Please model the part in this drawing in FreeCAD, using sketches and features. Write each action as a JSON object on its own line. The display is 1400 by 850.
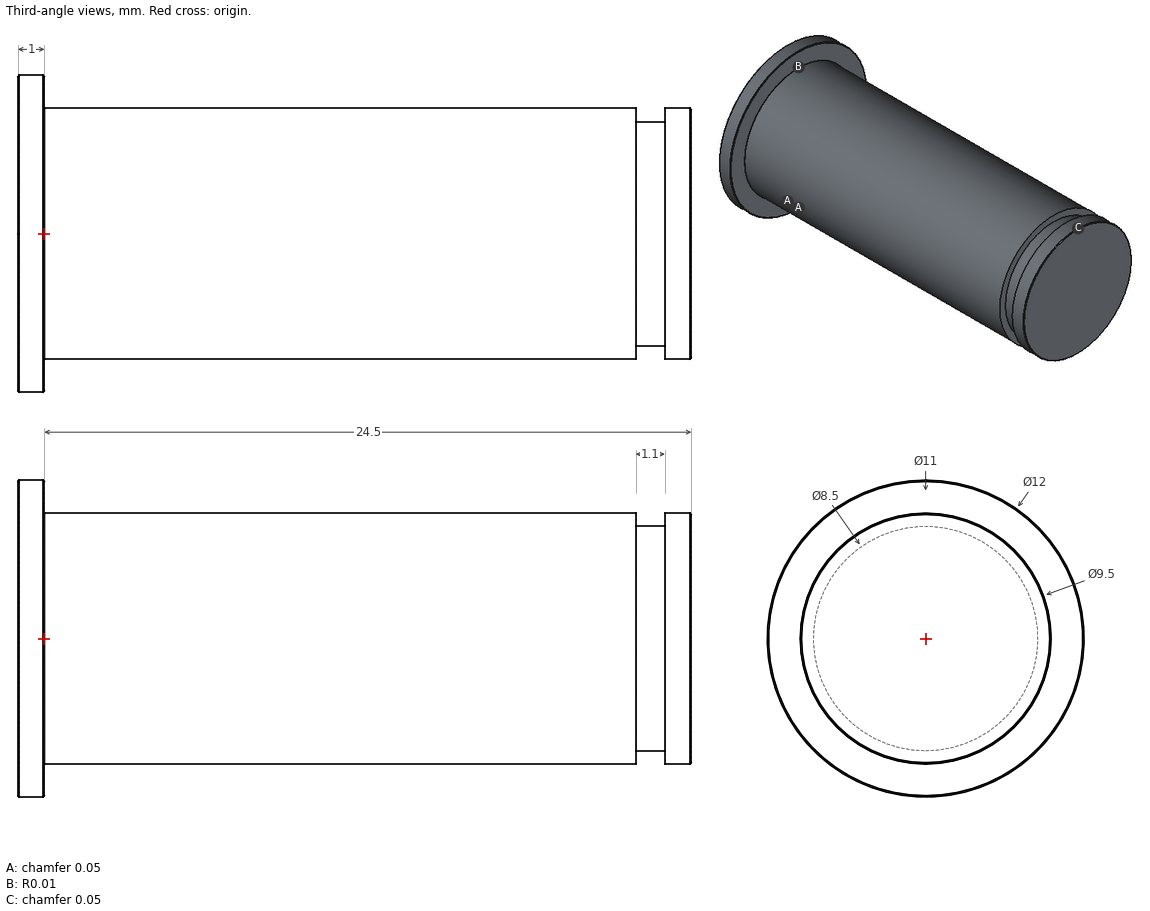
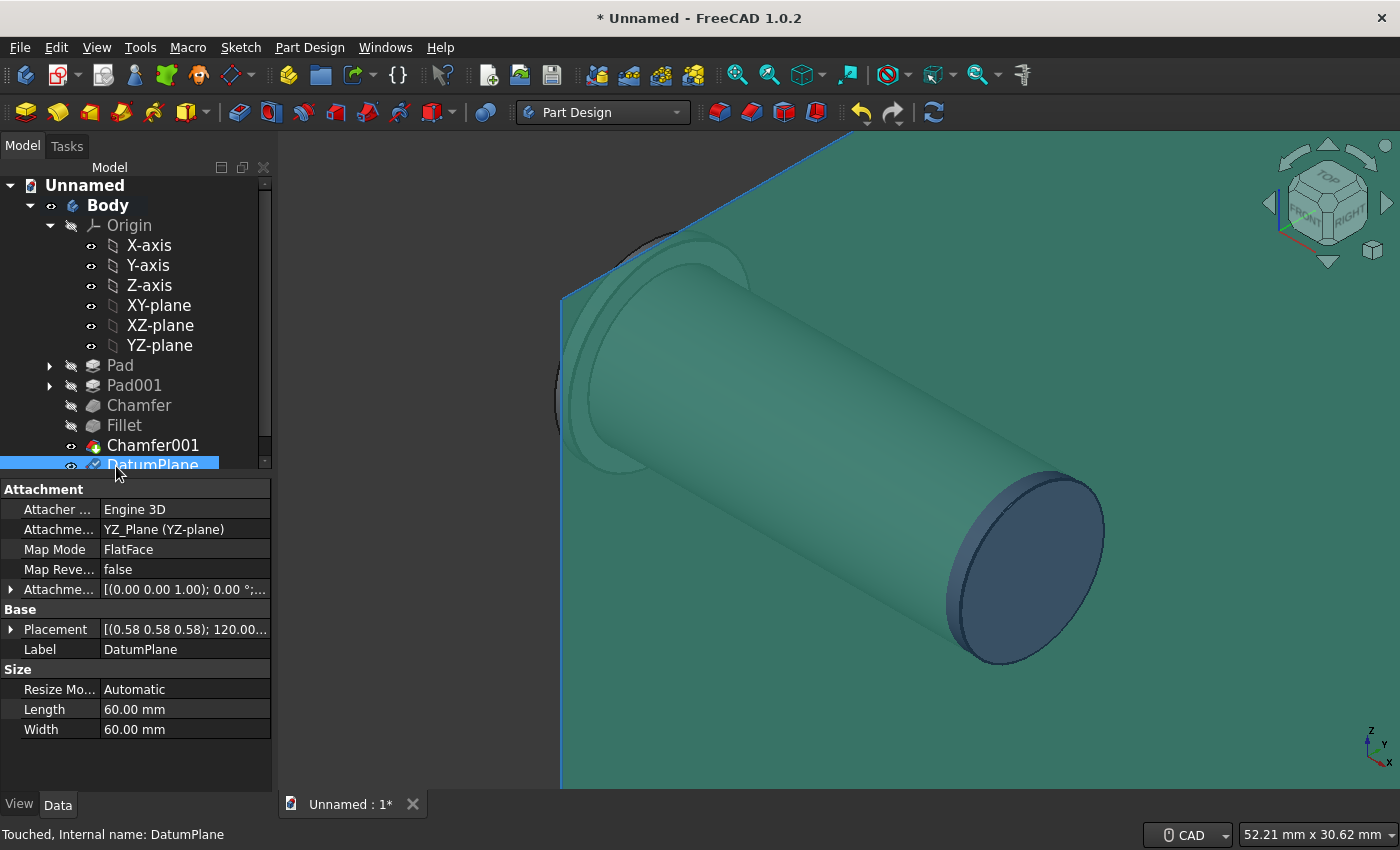
{"action": "left_click", "coordinate": [58, 76]}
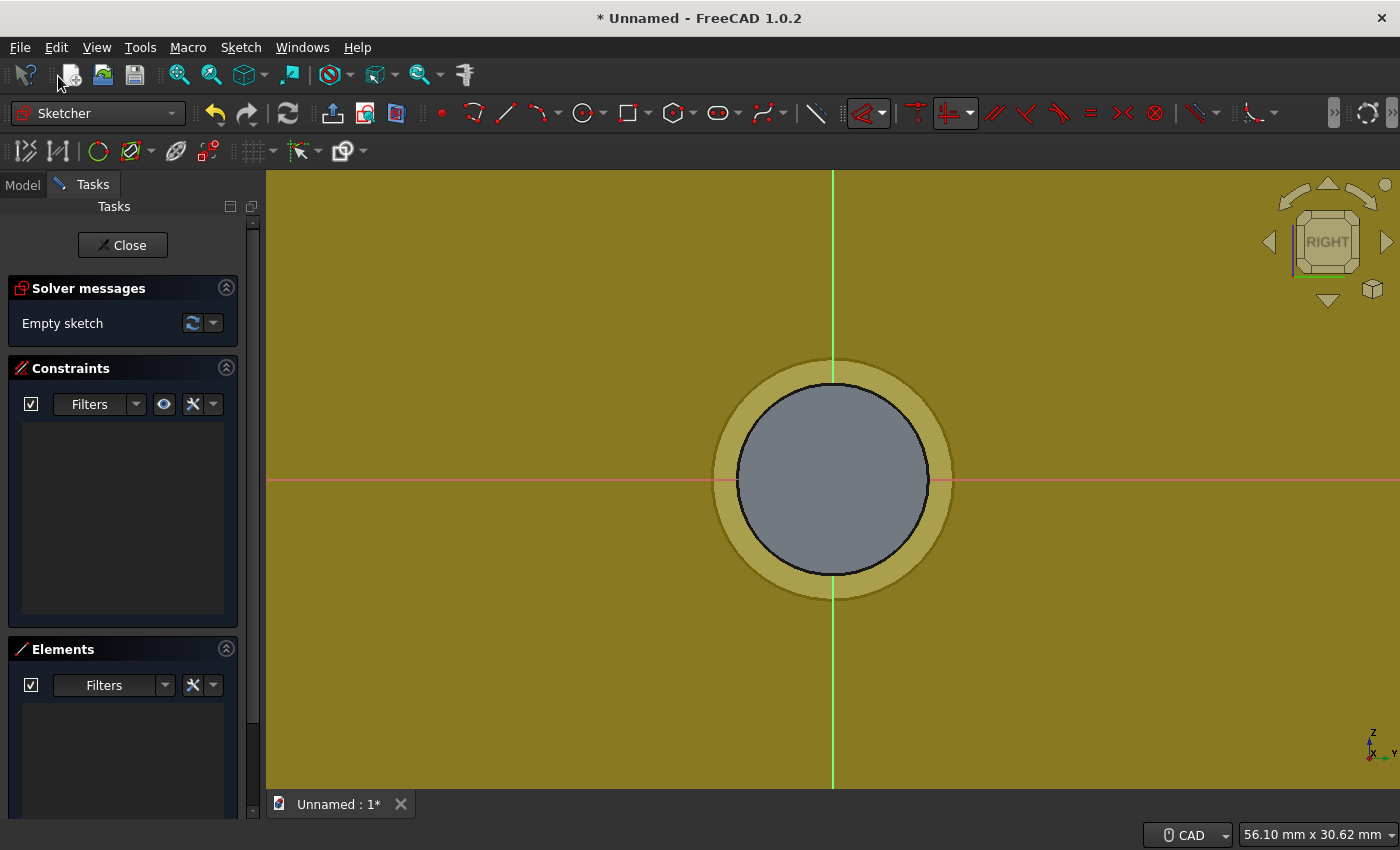
{"action": "left_click", "coordinate": [398, 114]}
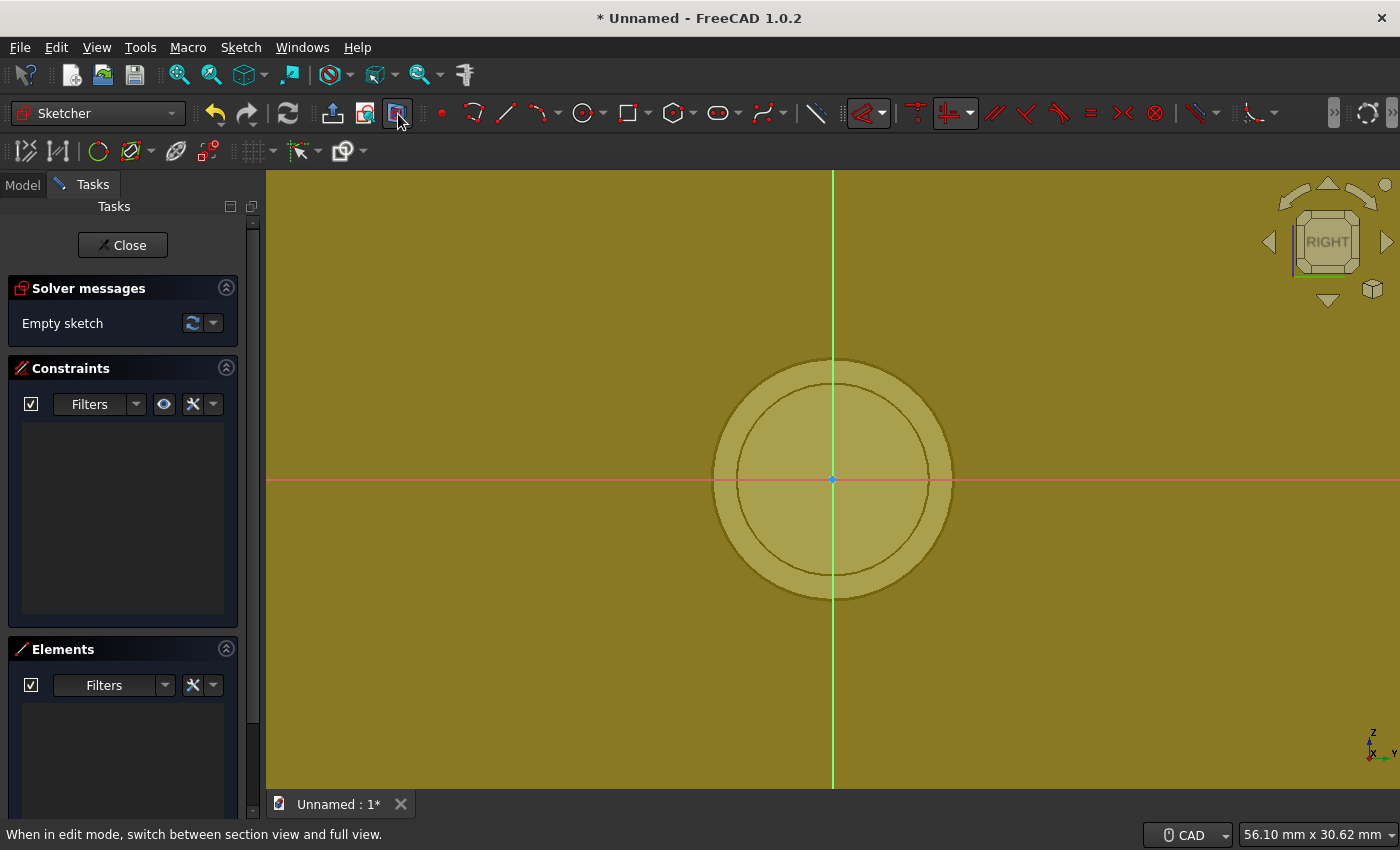
{"action": "scroll", "coordinate": [916, 480], "scroll_direction": "up", "scroll_amount": 3}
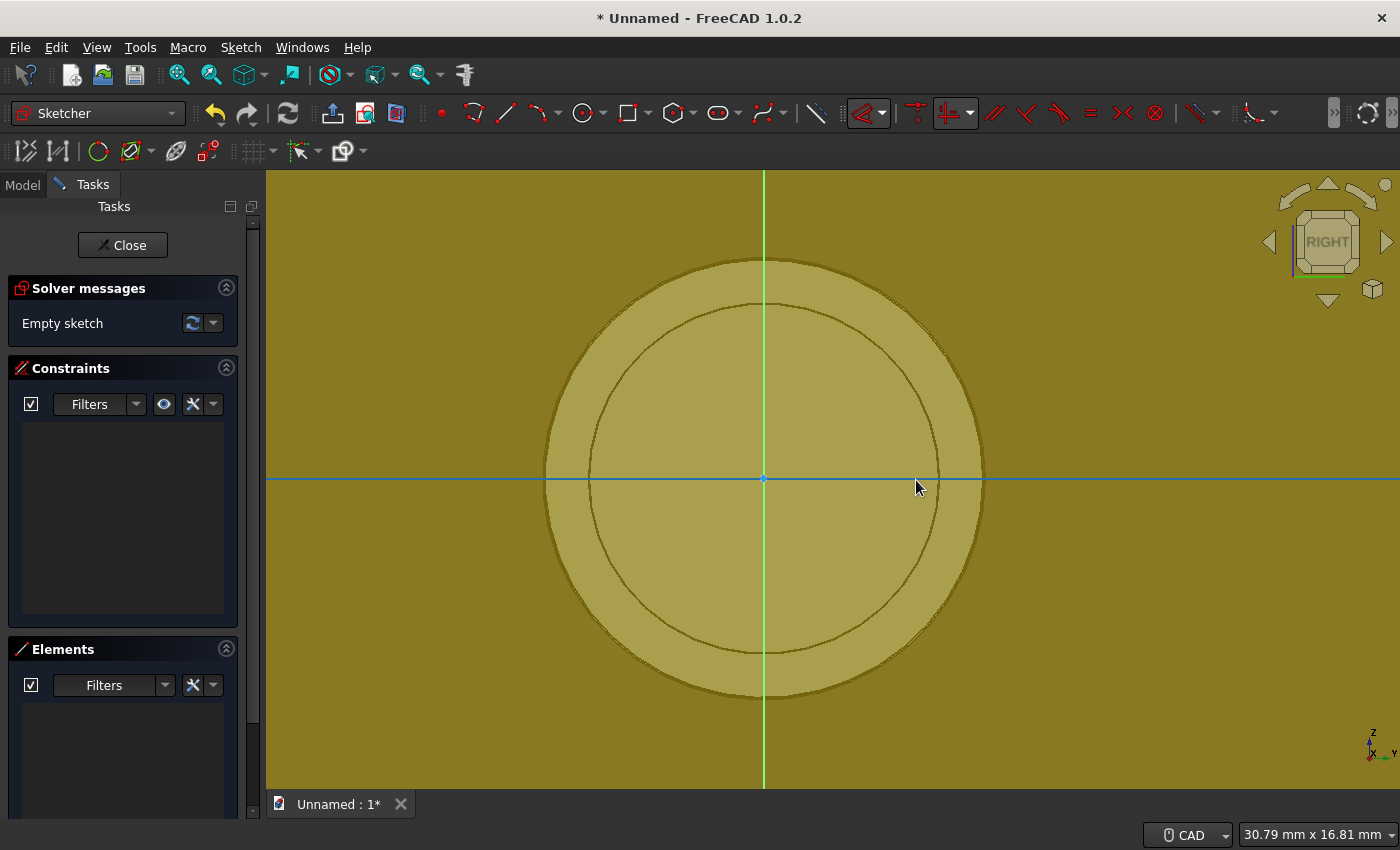
{"action": "left_click", "coordinate": [584, 114]}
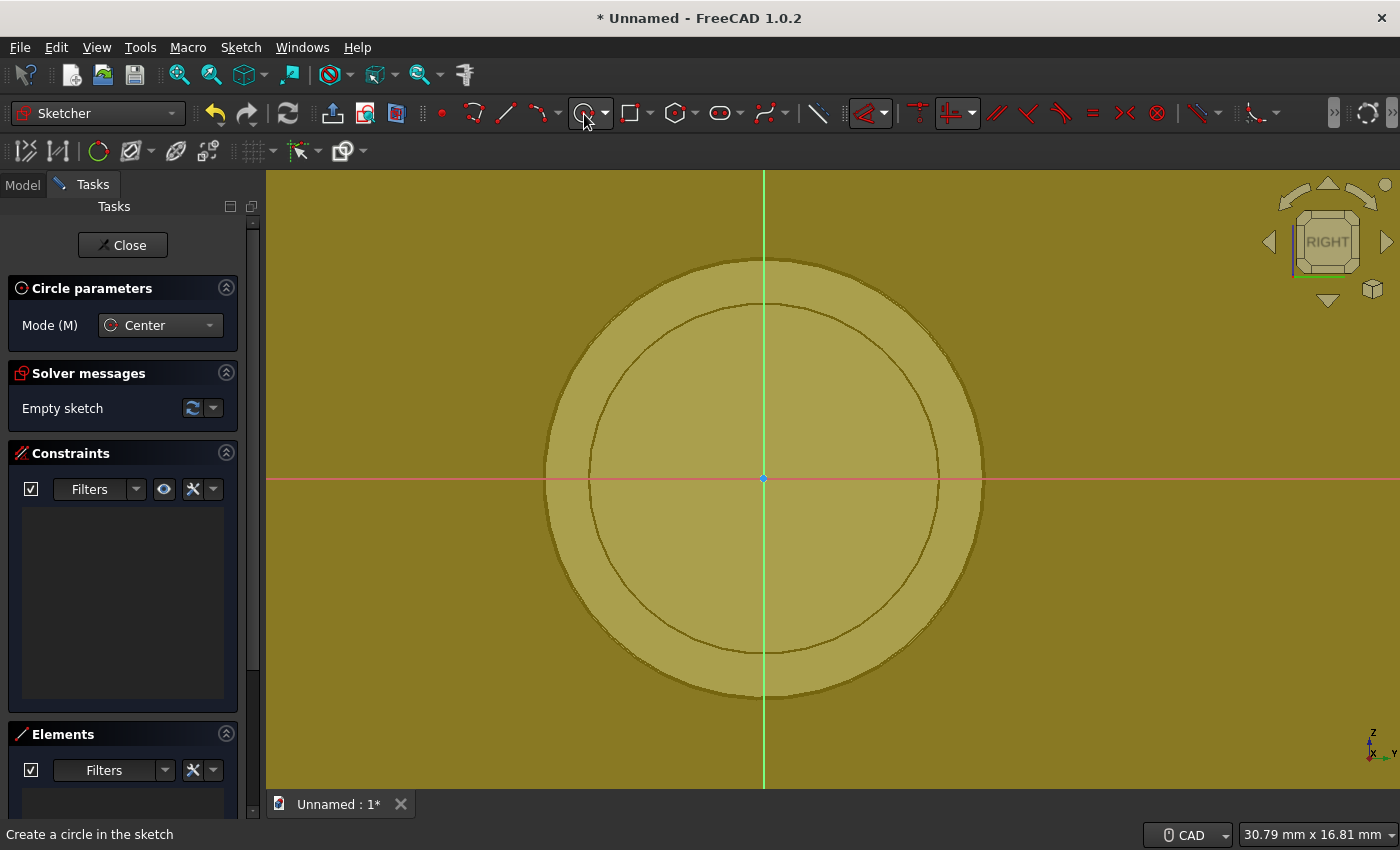
{"action": "left_click", "coordinate": [764, 479]}
{"action": "left_click", "coordinate": [907, 335]}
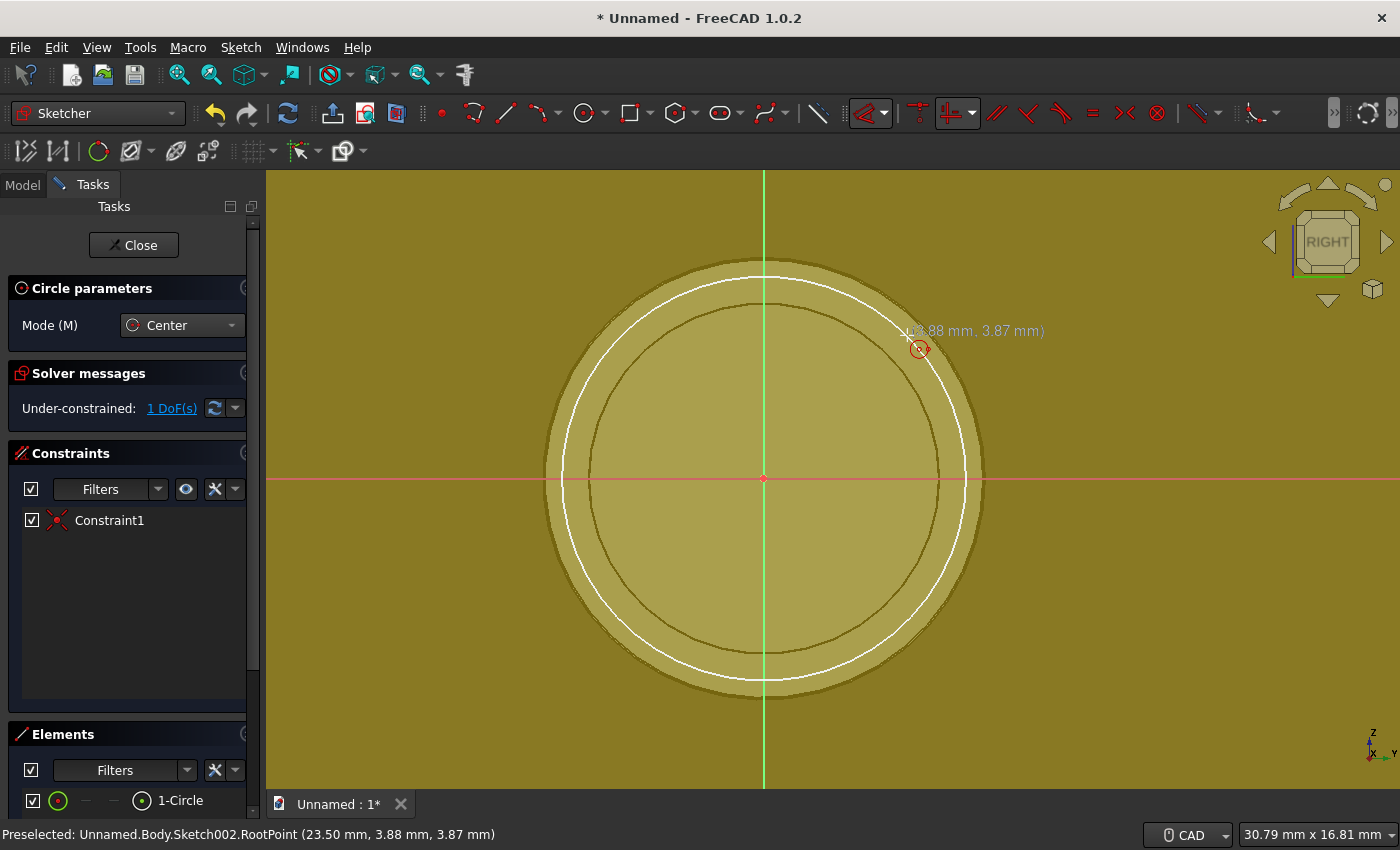
{"action": "left_click", "coordinate": [764, 479]}
{"action": "left_click", "coordinate": [875, 368]}
{"action": "key", "text": "Escape"}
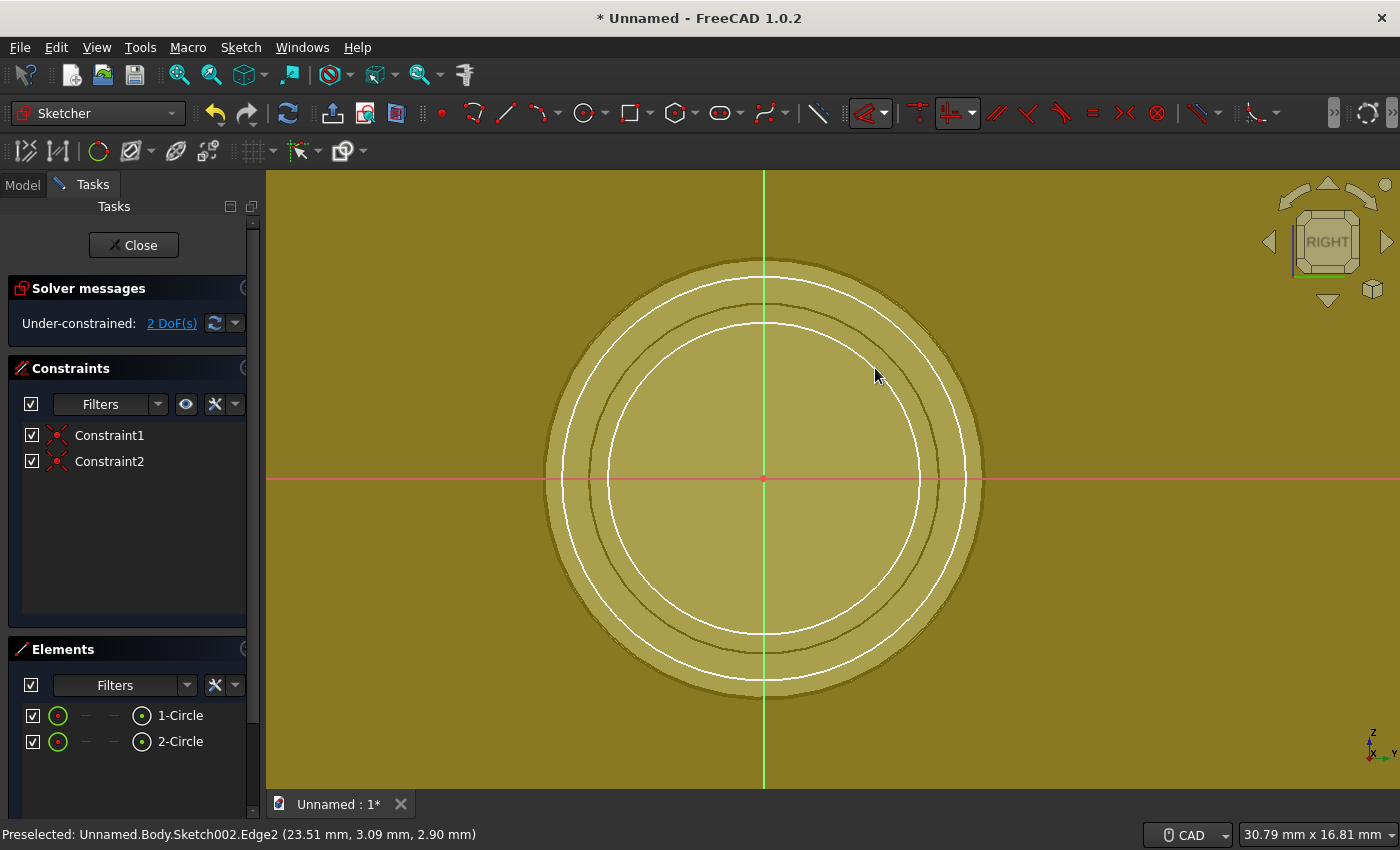
{"action": "key", "text": "d"}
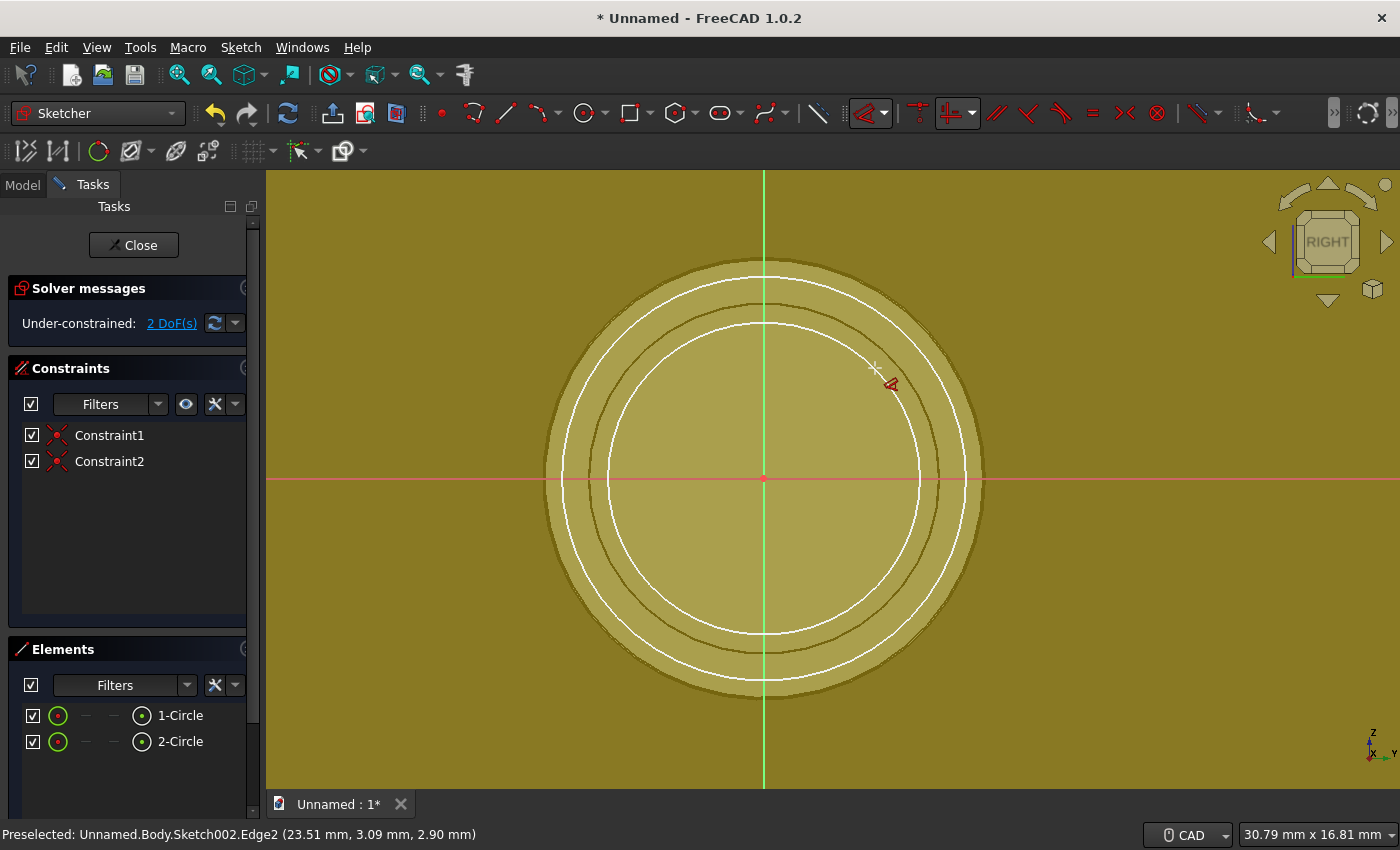
{"action": "left_click", "coordinate": [906, 335]}
{"action": "left_click", "coordinate": [928, 312]}